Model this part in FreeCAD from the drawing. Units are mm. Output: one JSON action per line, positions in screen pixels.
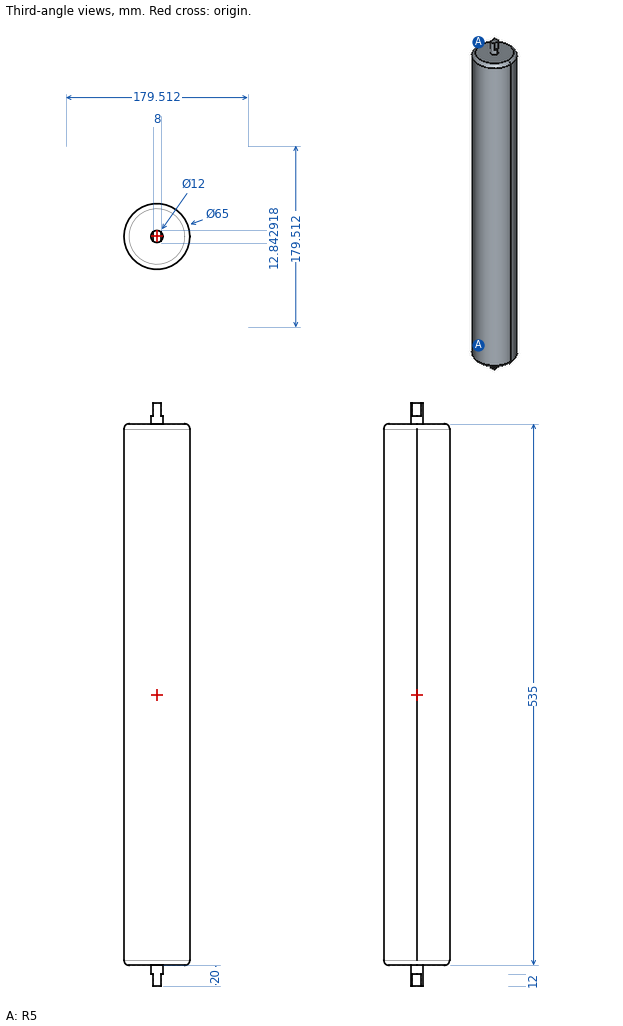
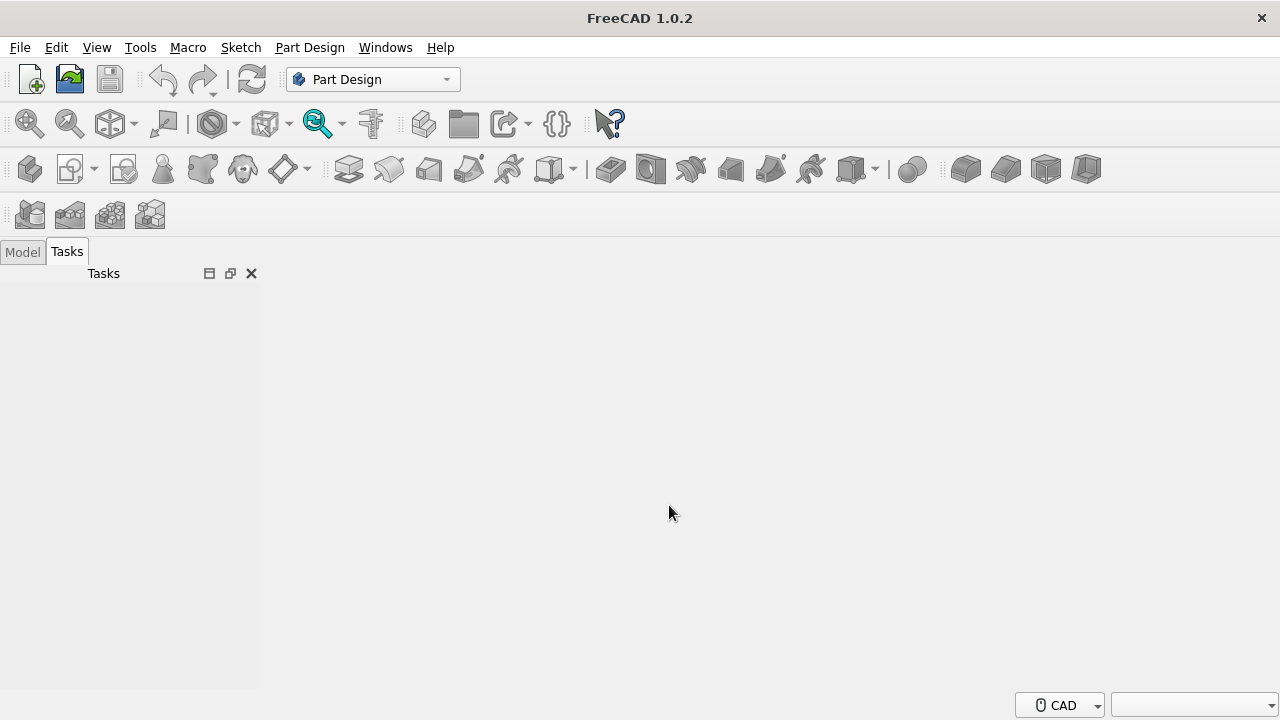
{"action": "left_click", "coordinate": [30, 80]}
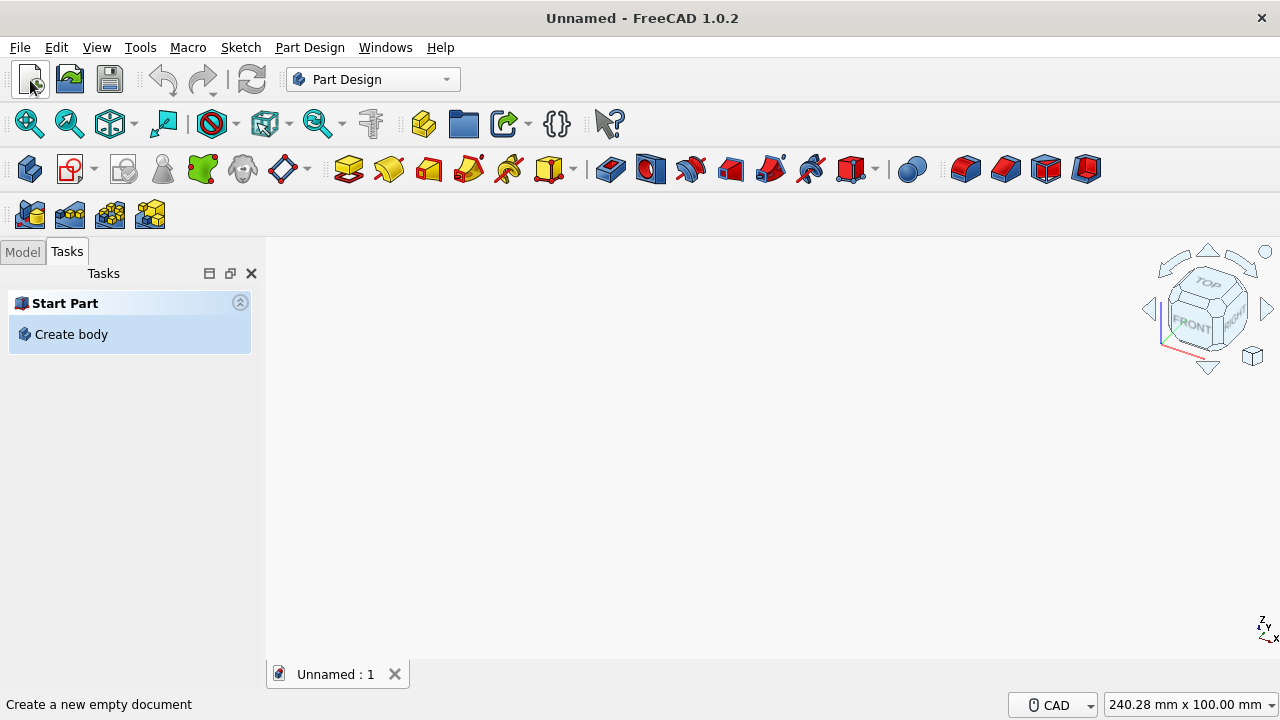
{"action": "left_click", "coordinate": [70, 170]}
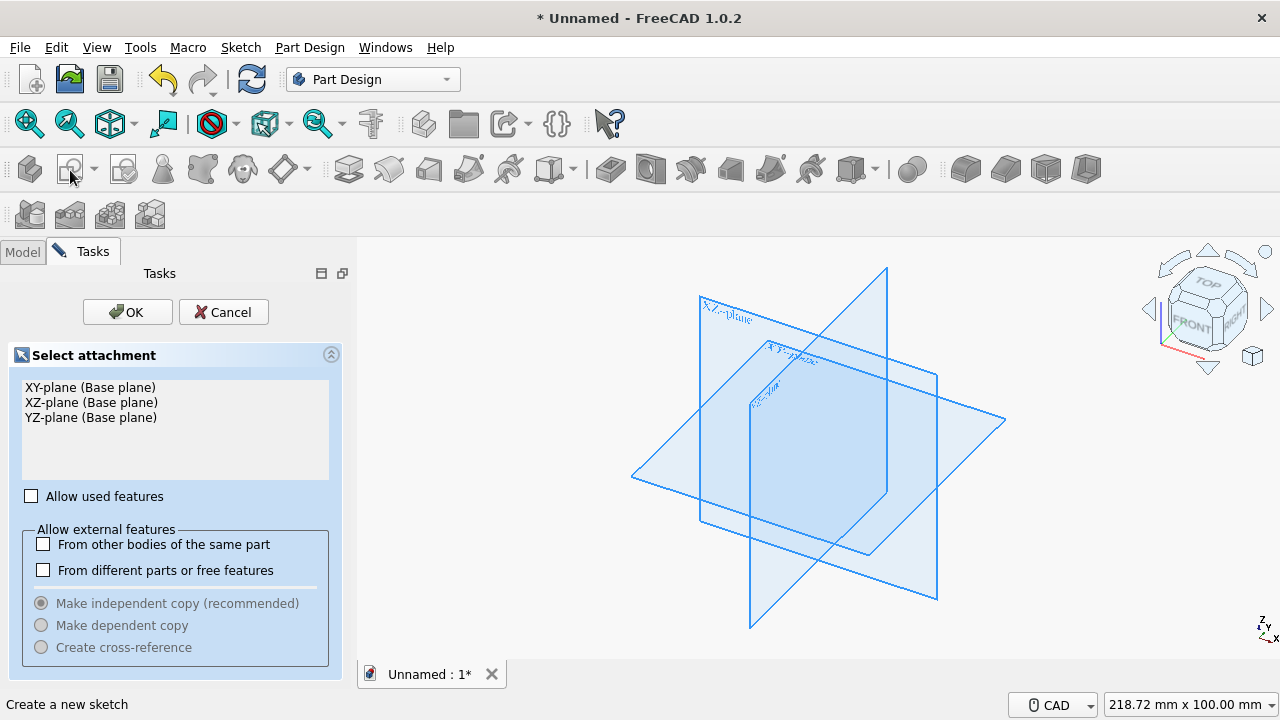
{"action": "left_click", "coordinate": [82, 388]}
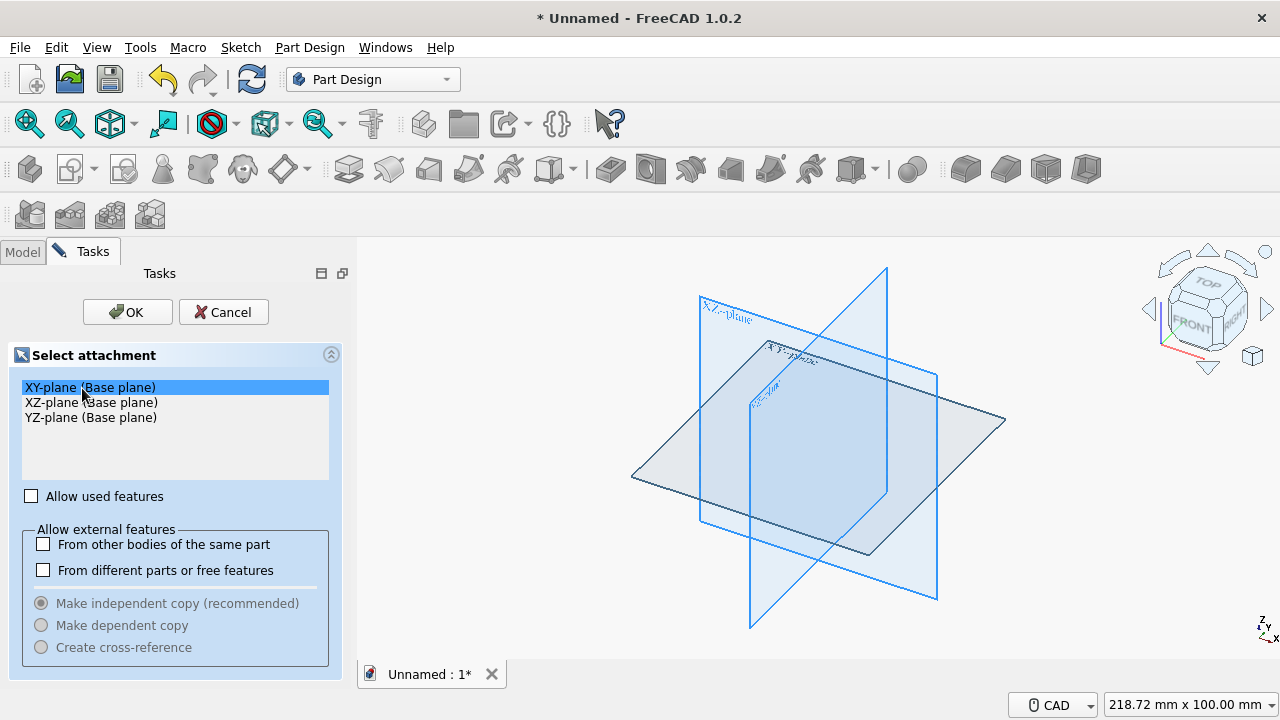
{"action": "left_click", "coordinate": [128, 312]}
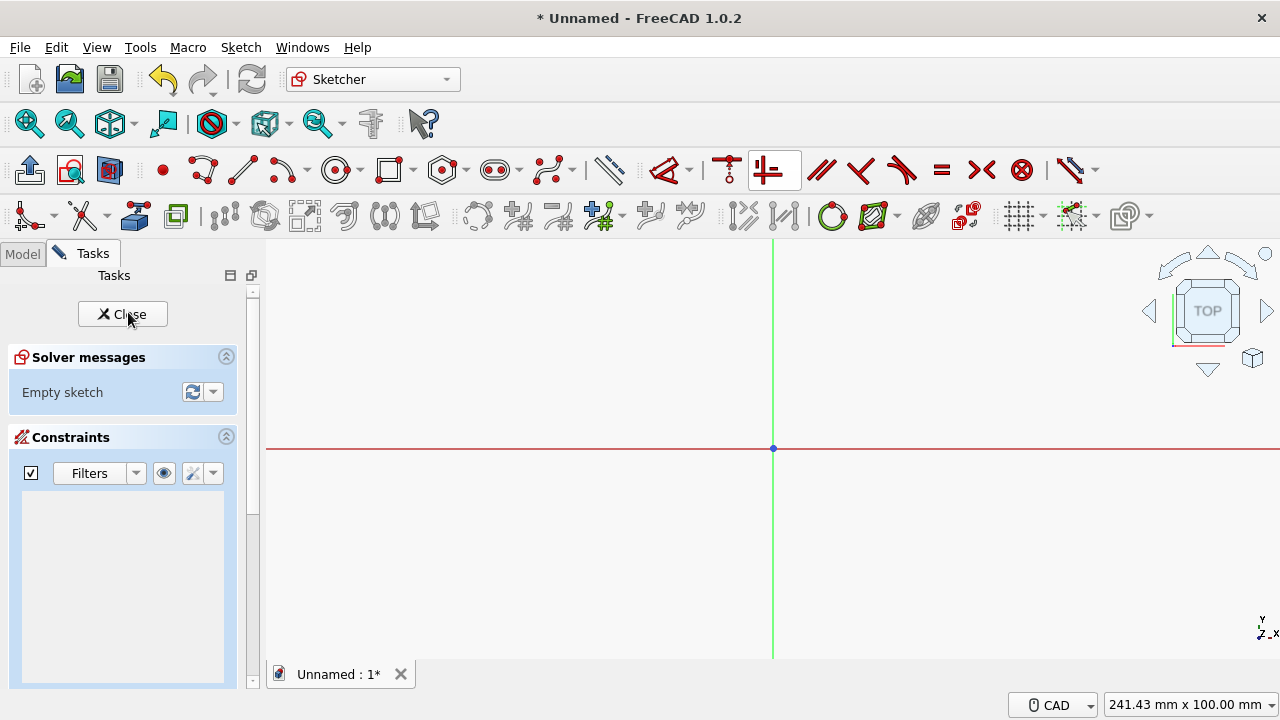
{"action": "left_click", "coordinate": [336, 170]}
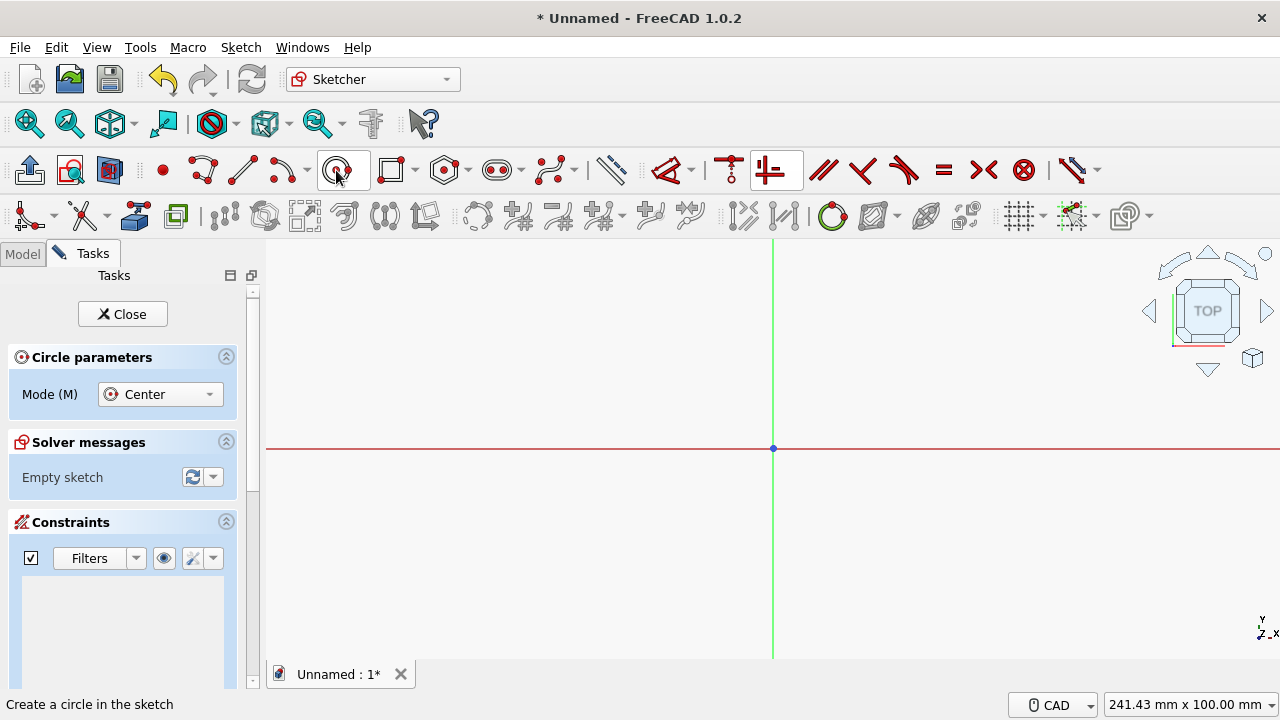
{"action": "left_click", "coordinate": [773, 449]}
{"action": "left_click", "coordinate": [870, 352]}
{"action": "key", "text": "Escape"}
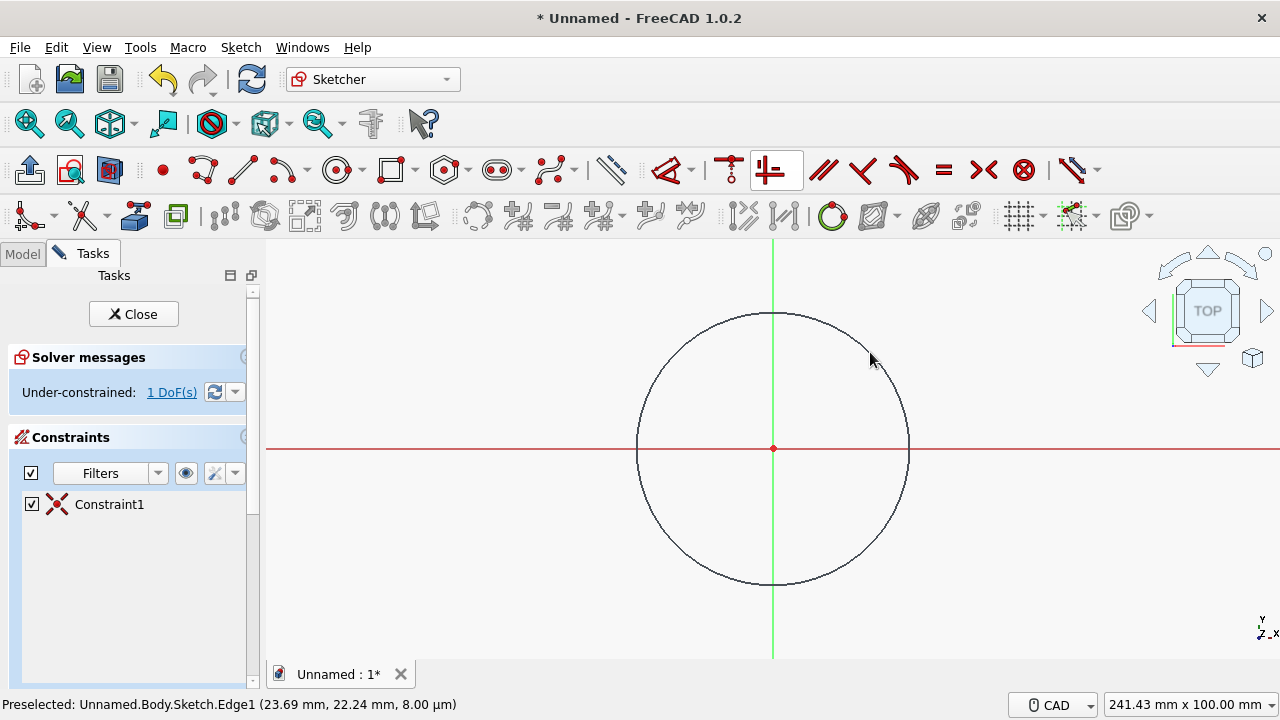
{"action": "left_click", "coordinate": [869, 352]}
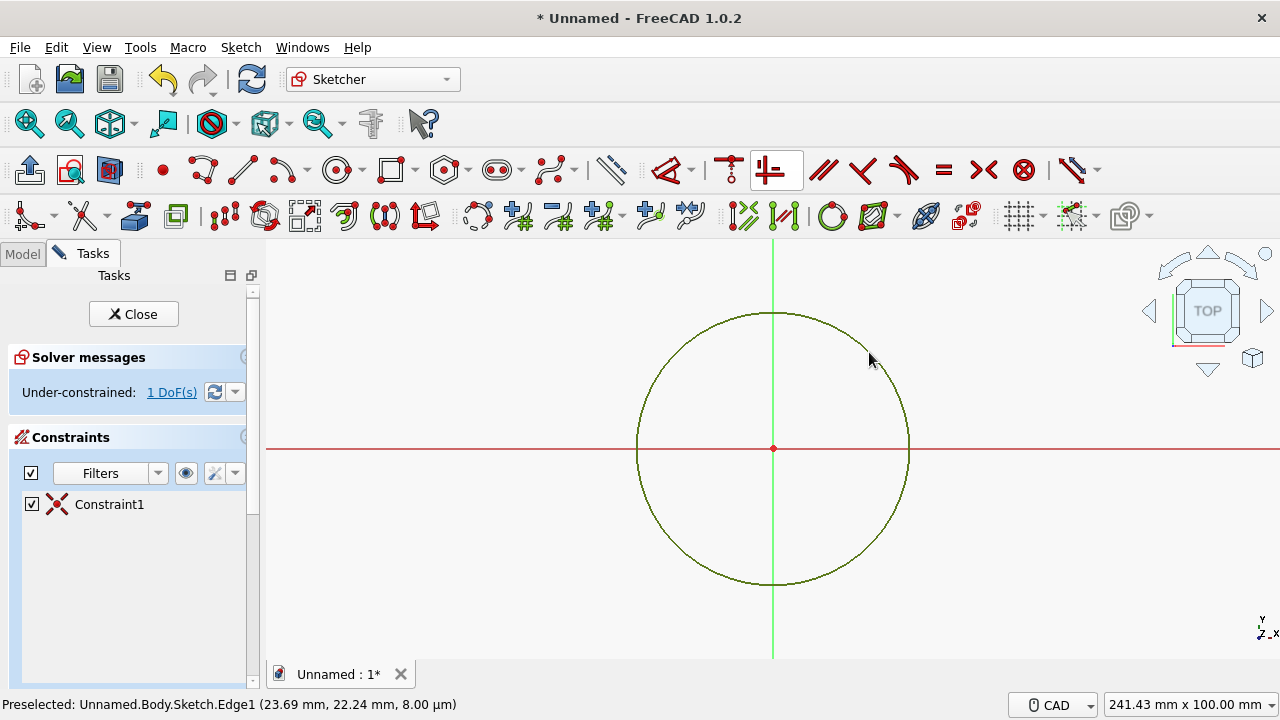
{"action": "key", "text": "k o"}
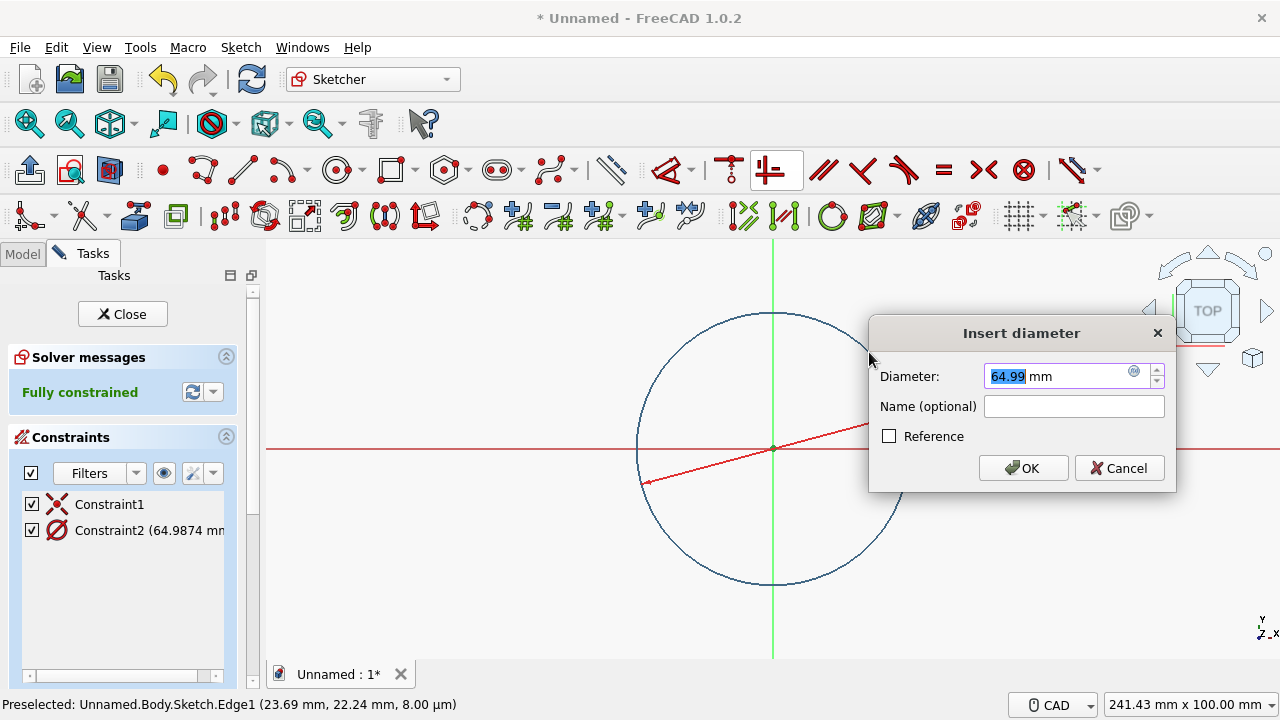
{"action": "type", "text": "65"}
{"action": "key", "text": "Return"}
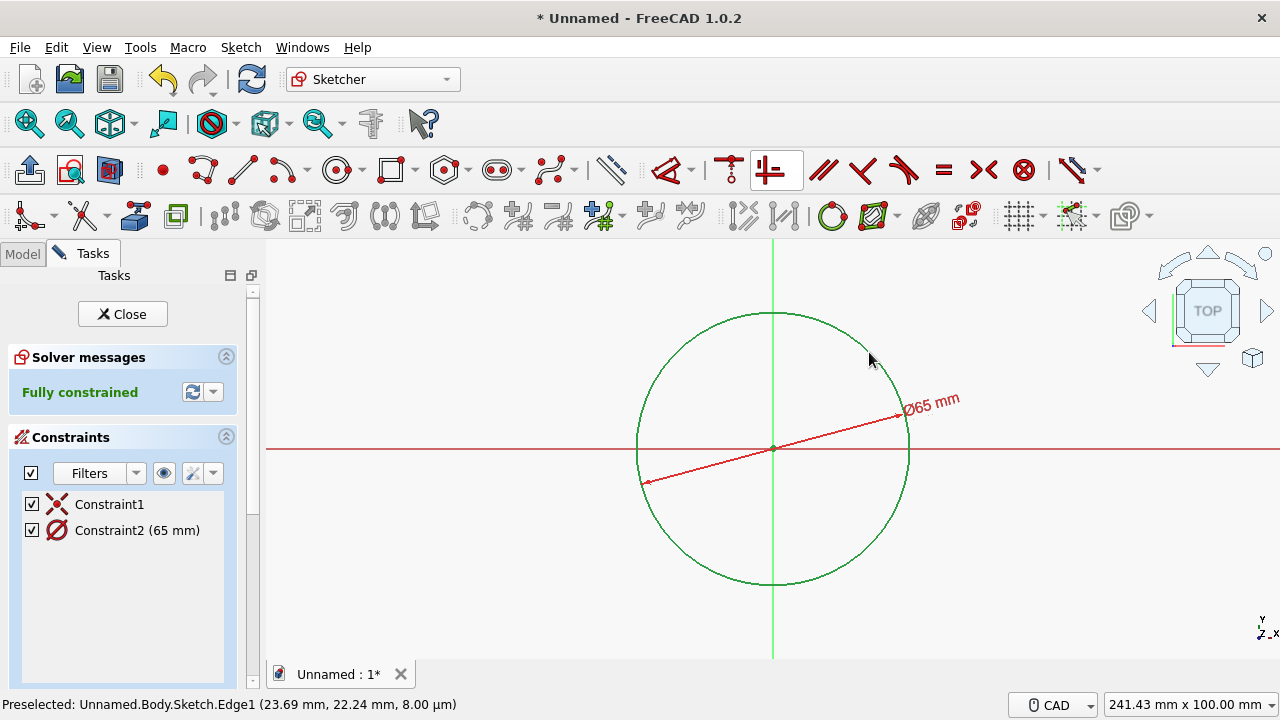
{"action": "left_click", "coordinate": [123, 314]}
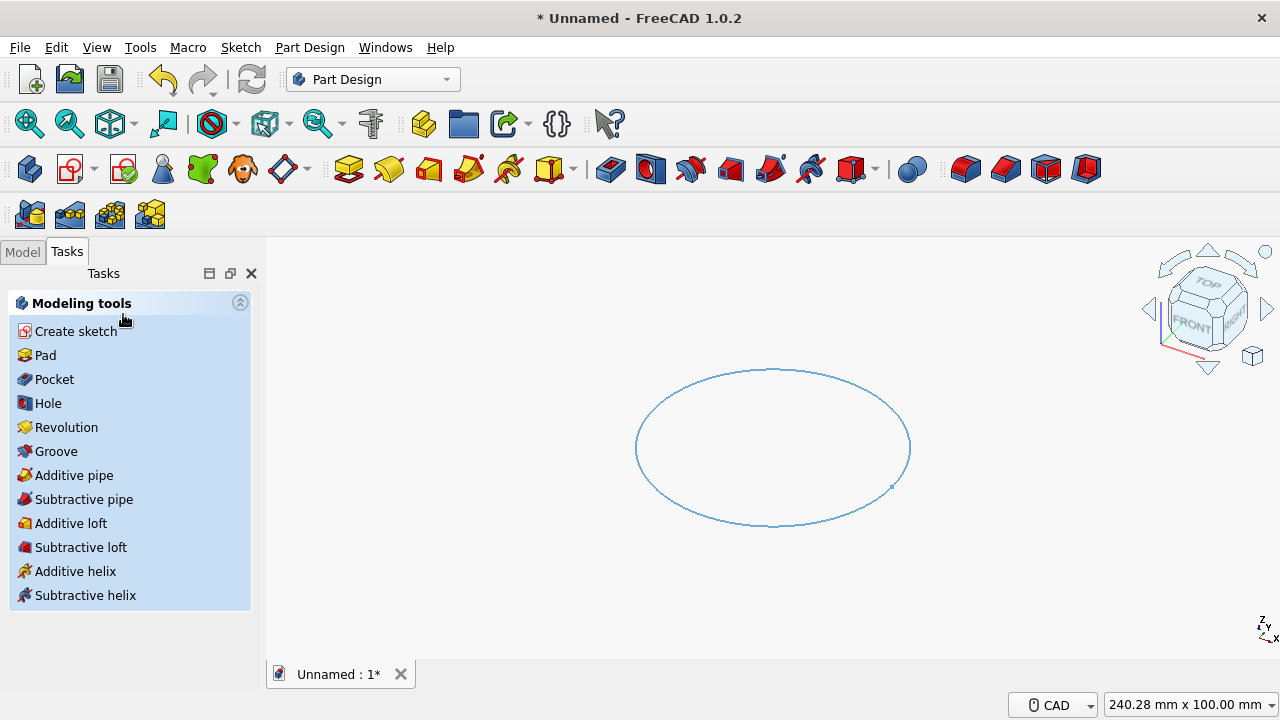
{"action": "left_click", "coordinate": [350, 170]}